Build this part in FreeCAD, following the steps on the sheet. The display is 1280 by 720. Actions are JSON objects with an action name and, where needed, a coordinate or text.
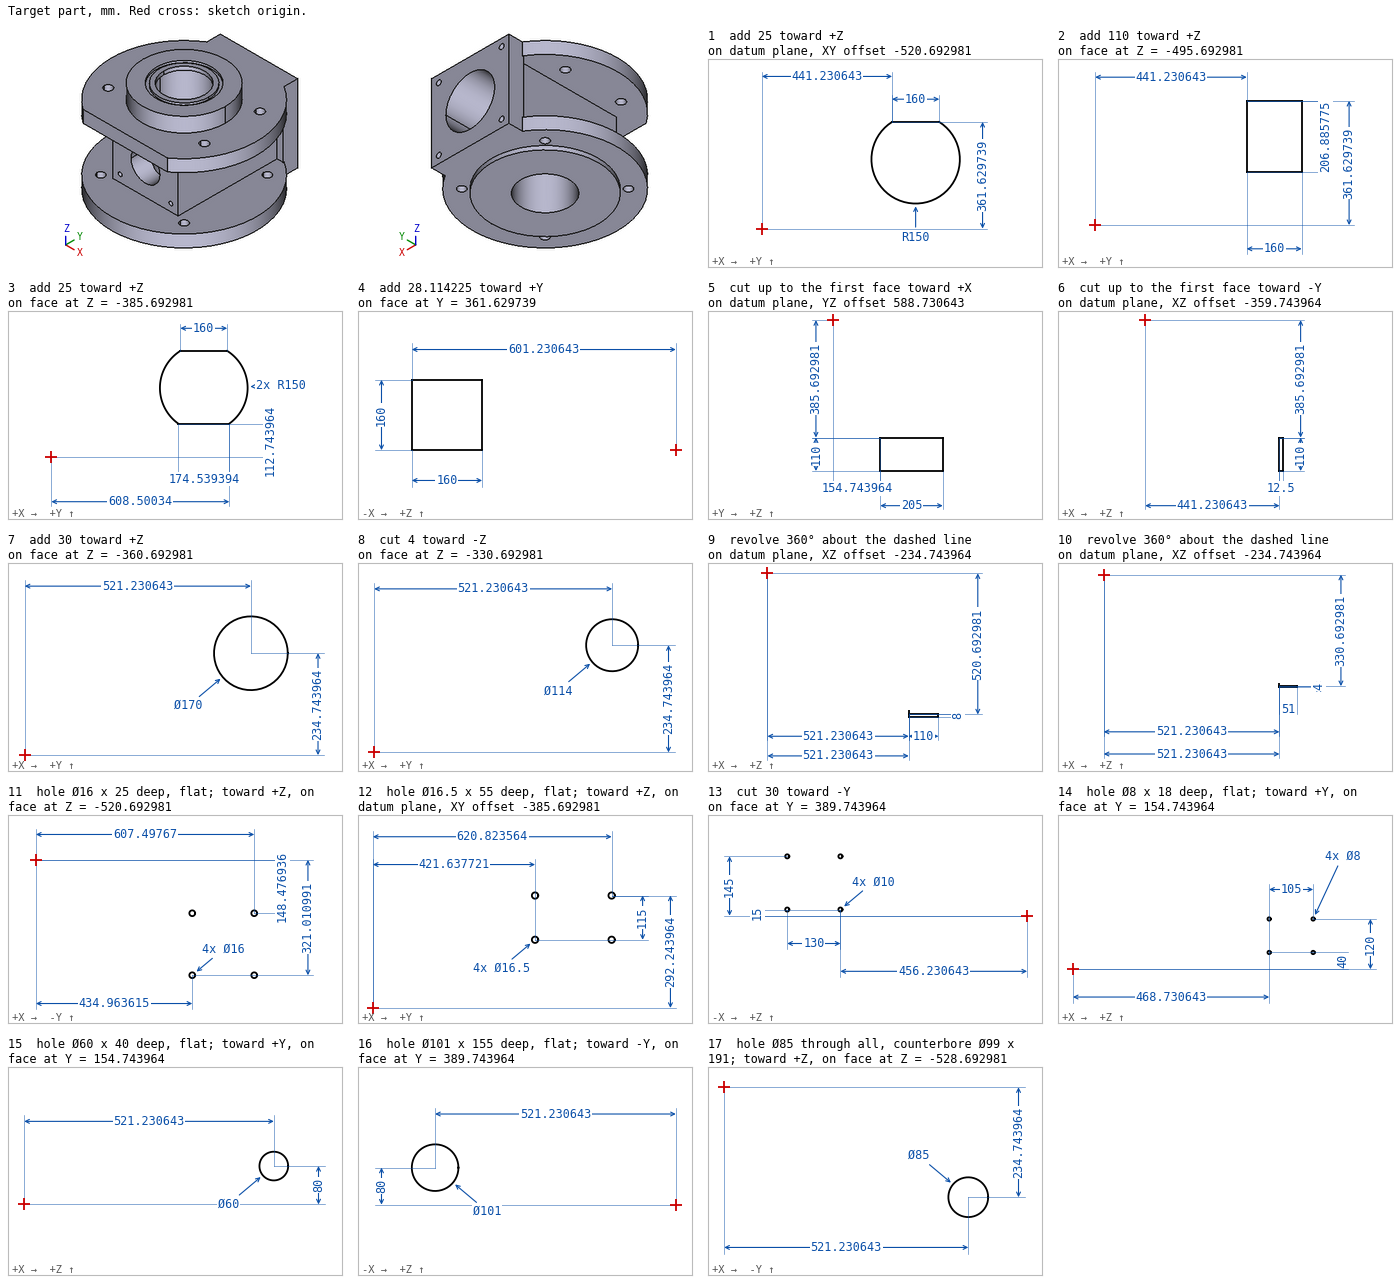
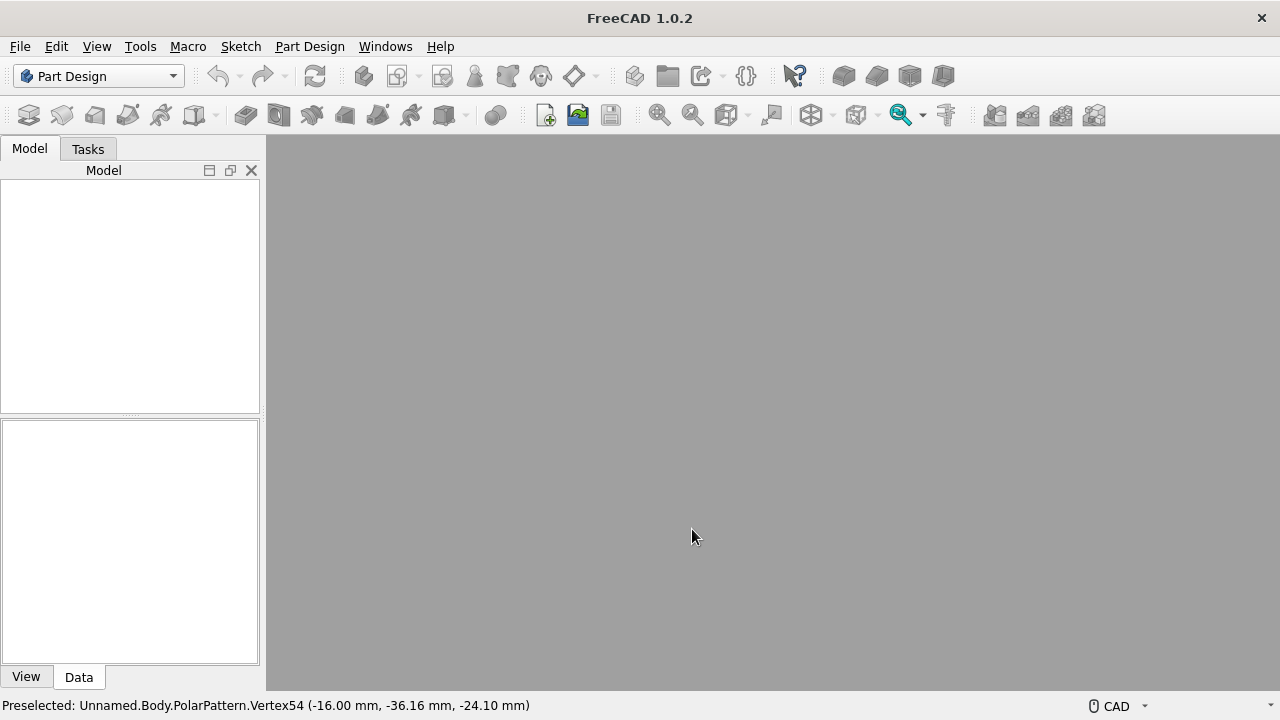
{"action": "left_click", "coordinate": [545, 116]}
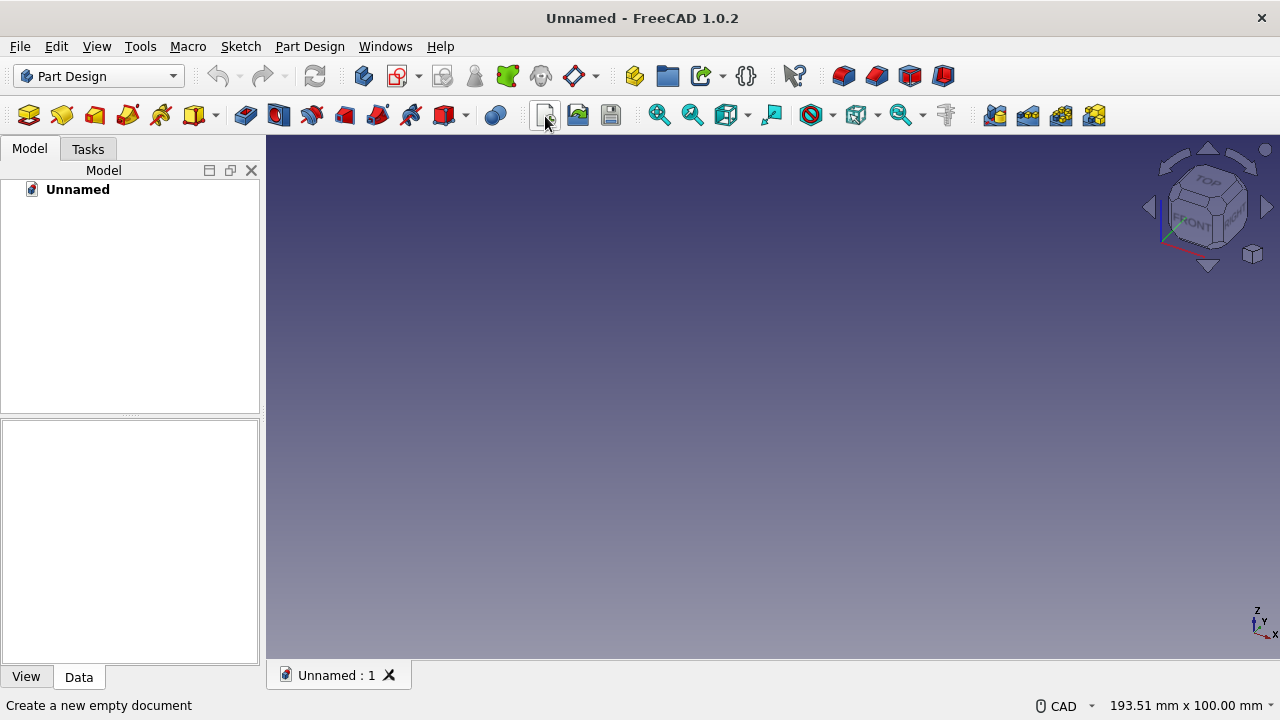
{"action": "left_click", "coordinate": [364, 76]}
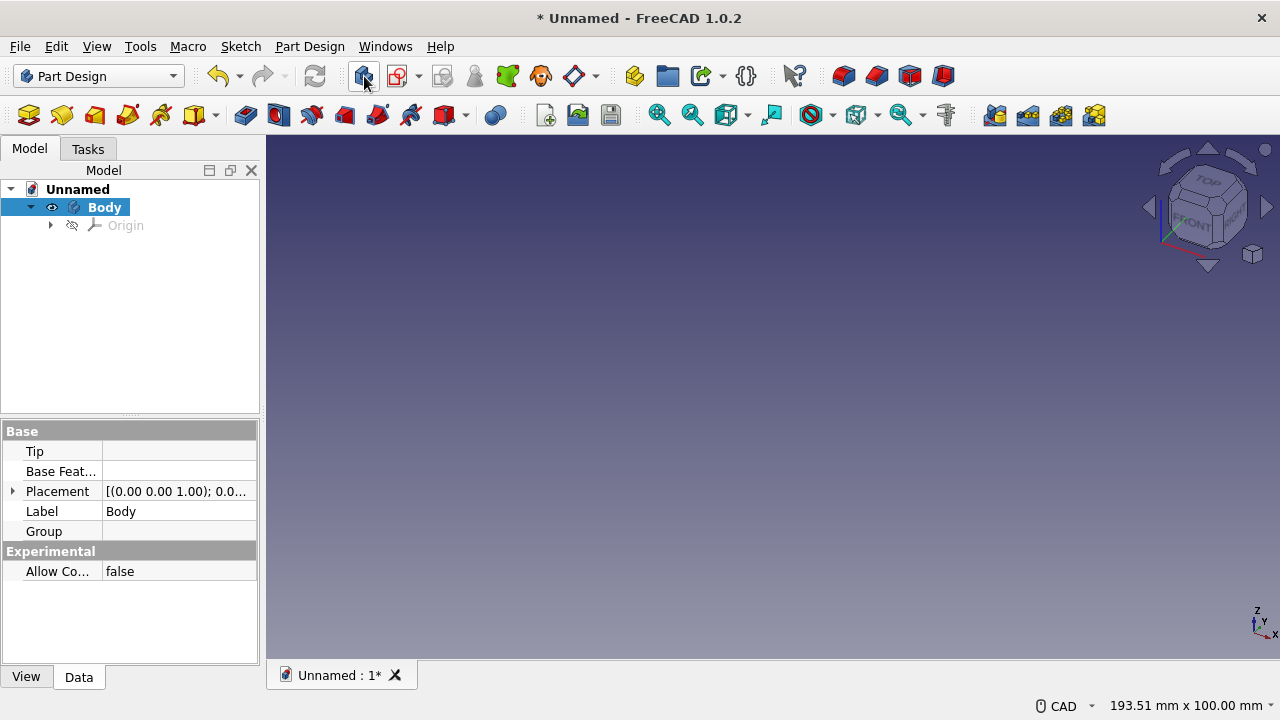
{"action": "left_click", "coordinate": [51, 225]}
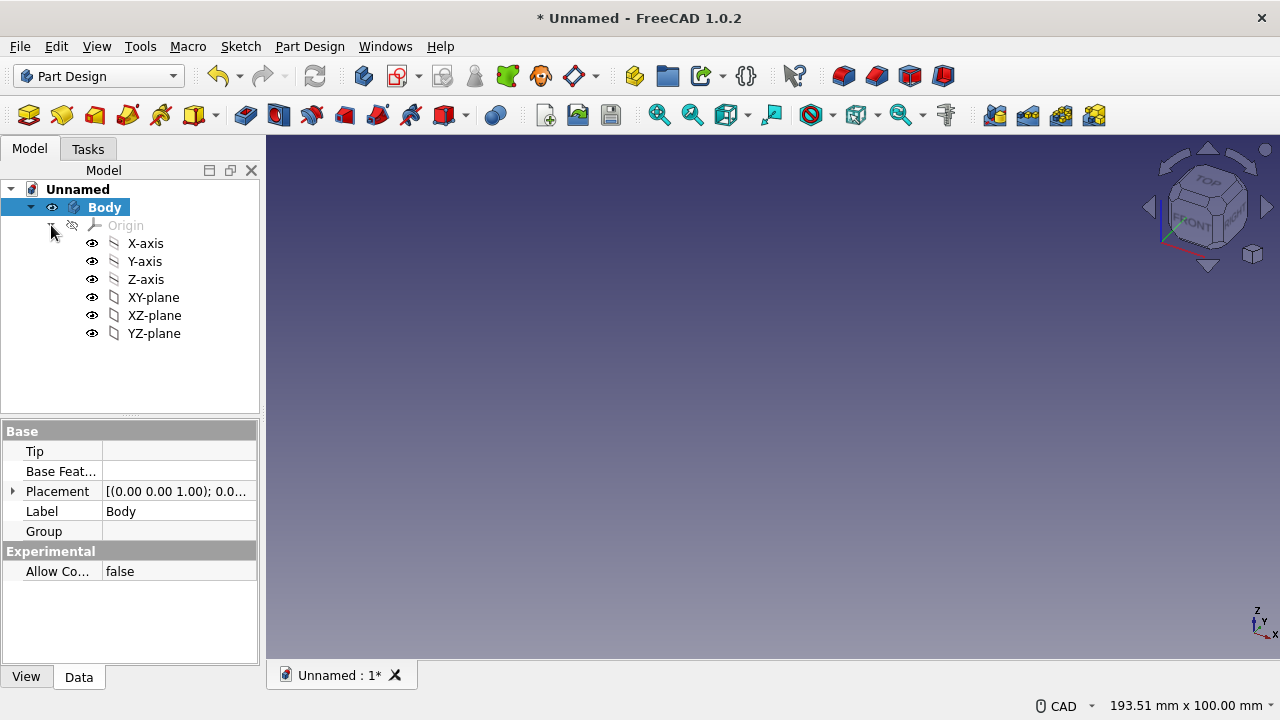
{"action": "left_click", "coordinate": [137, 297]}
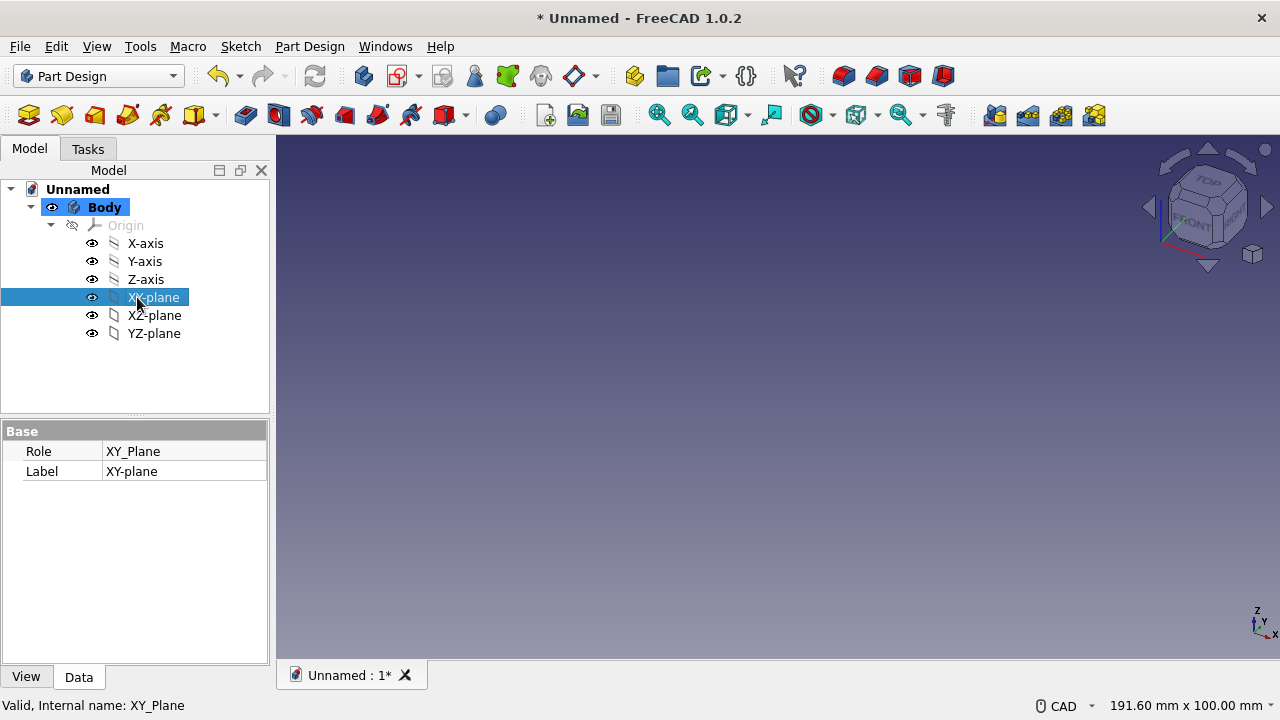
{"action": "left_click", "coordinate": [574, 76]}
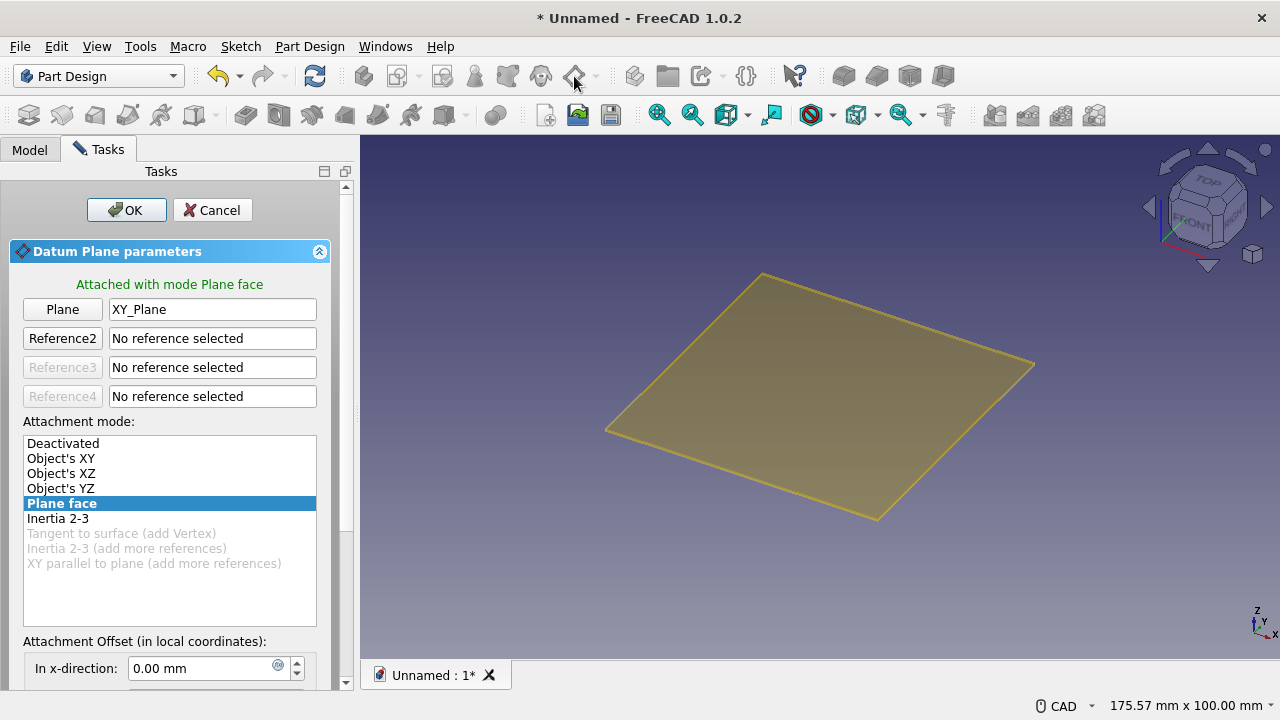
{"action": "scroll", "coordinate": [346, 436], "scroll_direction": "down", "scroll_amount": 2}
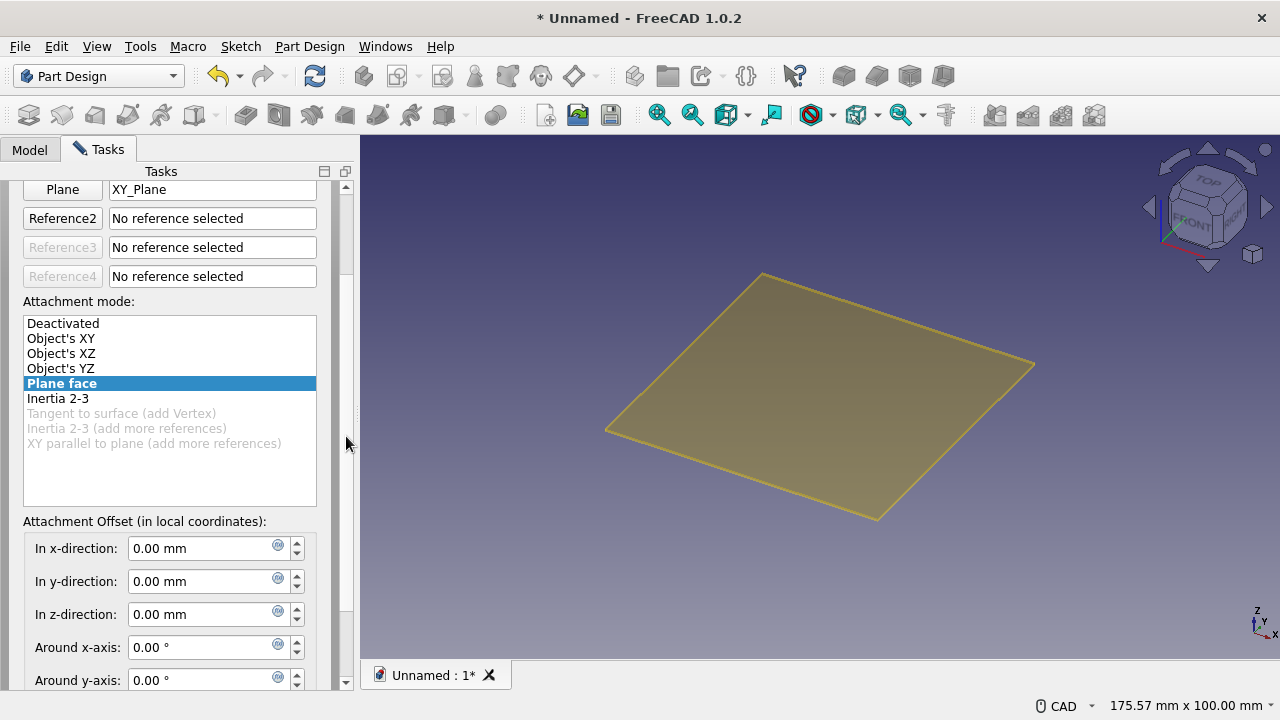
{"action": "triple_click", "coordinate": [210, 614]}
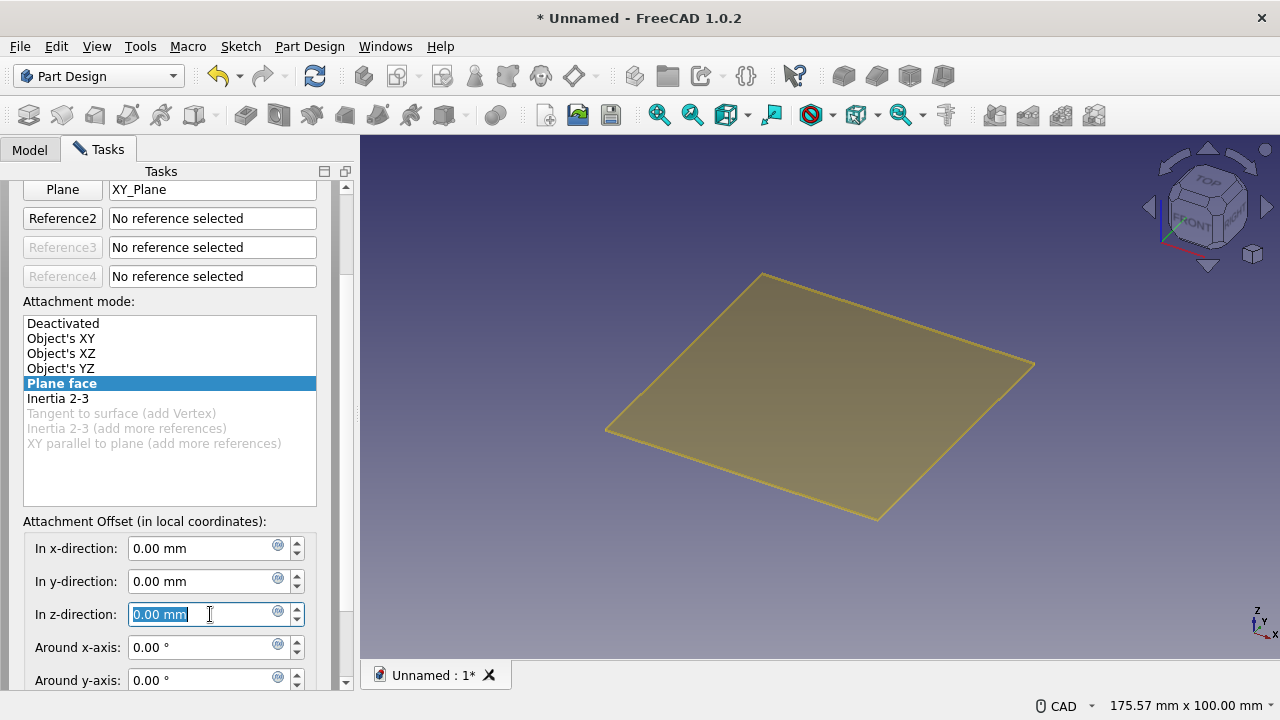
{"action": "type", "text": "-520.692981"}
{"action": "key", "text": "Tab"}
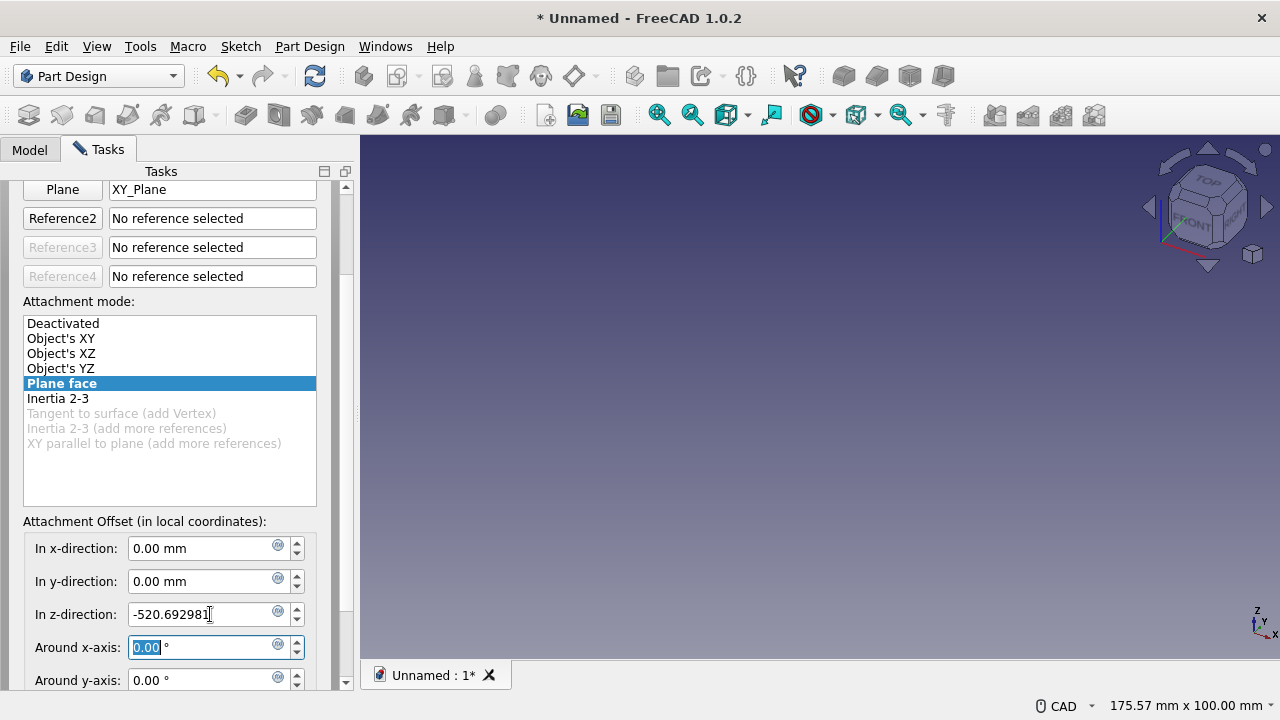
{"action": "scroll", "coordinate": [346, 436], "scroll_direction": "up", "scroll_amount": 3}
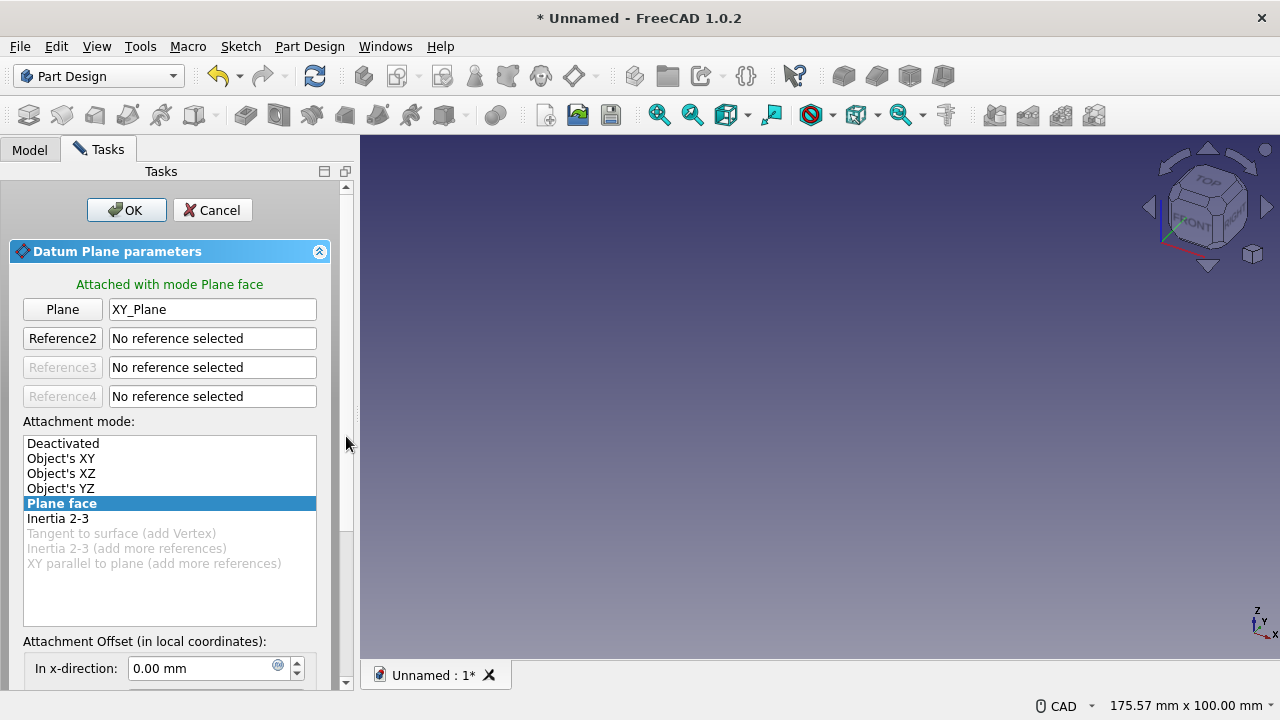
{"action": "left_click", "coordinate": [127, 210]}